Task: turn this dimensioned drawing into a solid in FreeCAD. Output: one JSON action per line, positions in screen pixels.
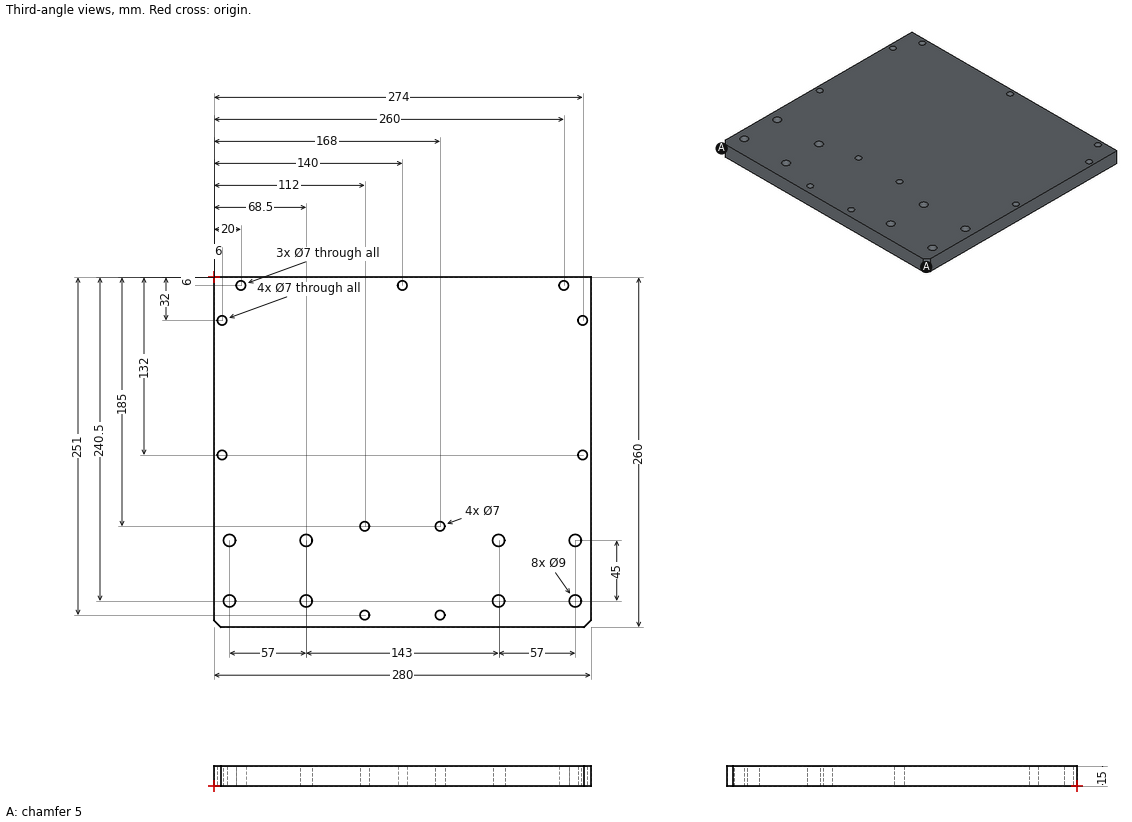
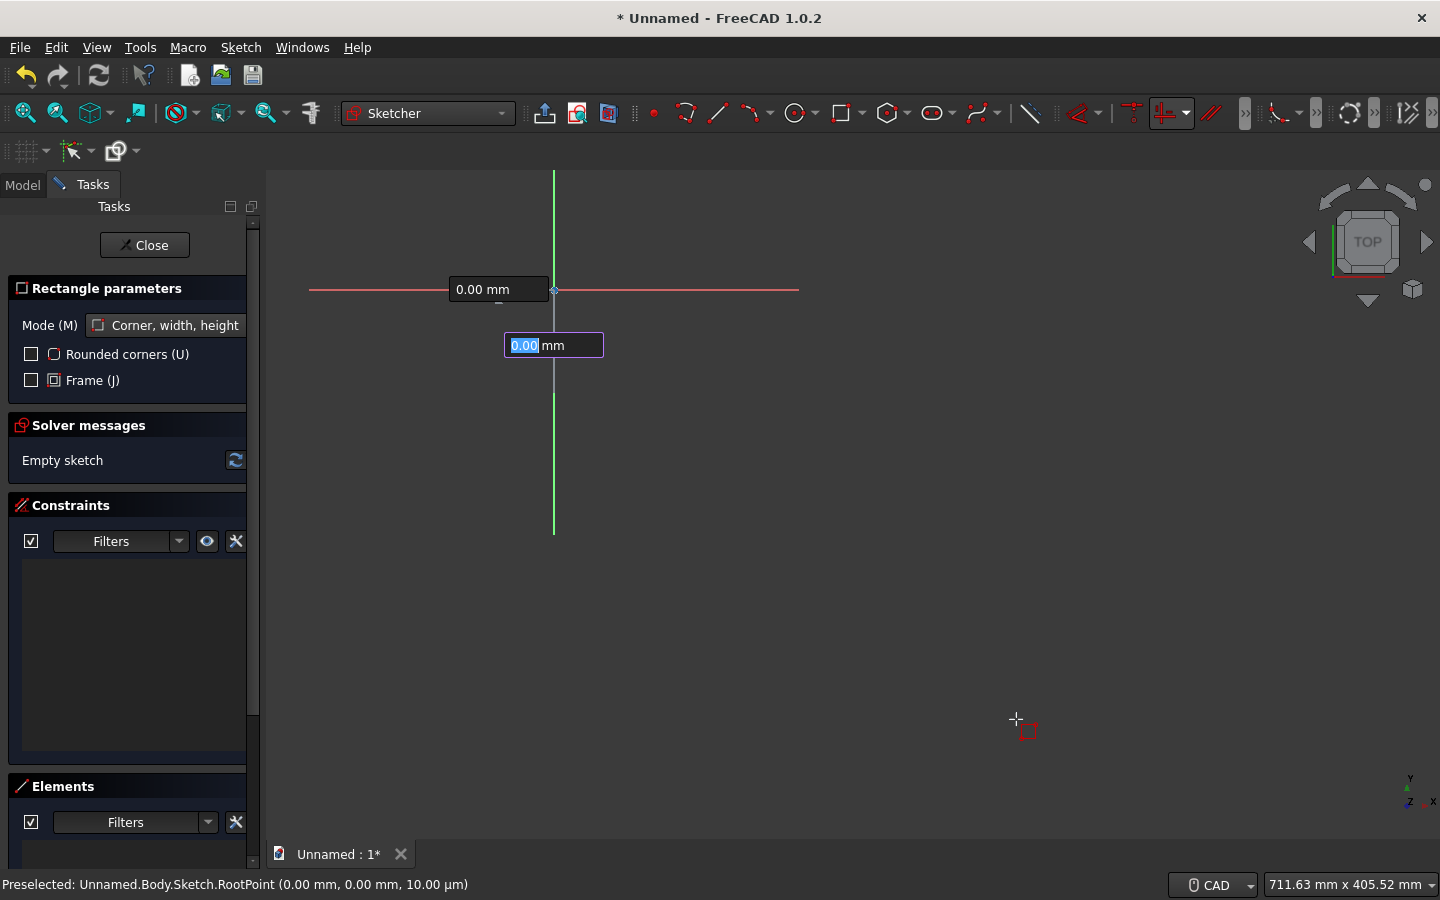
{"action": "type", "text": "280"}
{"action": "key", "text": "Tab"}
{"action": "type", "text": "260"}
{"action": "key", "text": "Return"}
{"action": "key", "text": "Escape"}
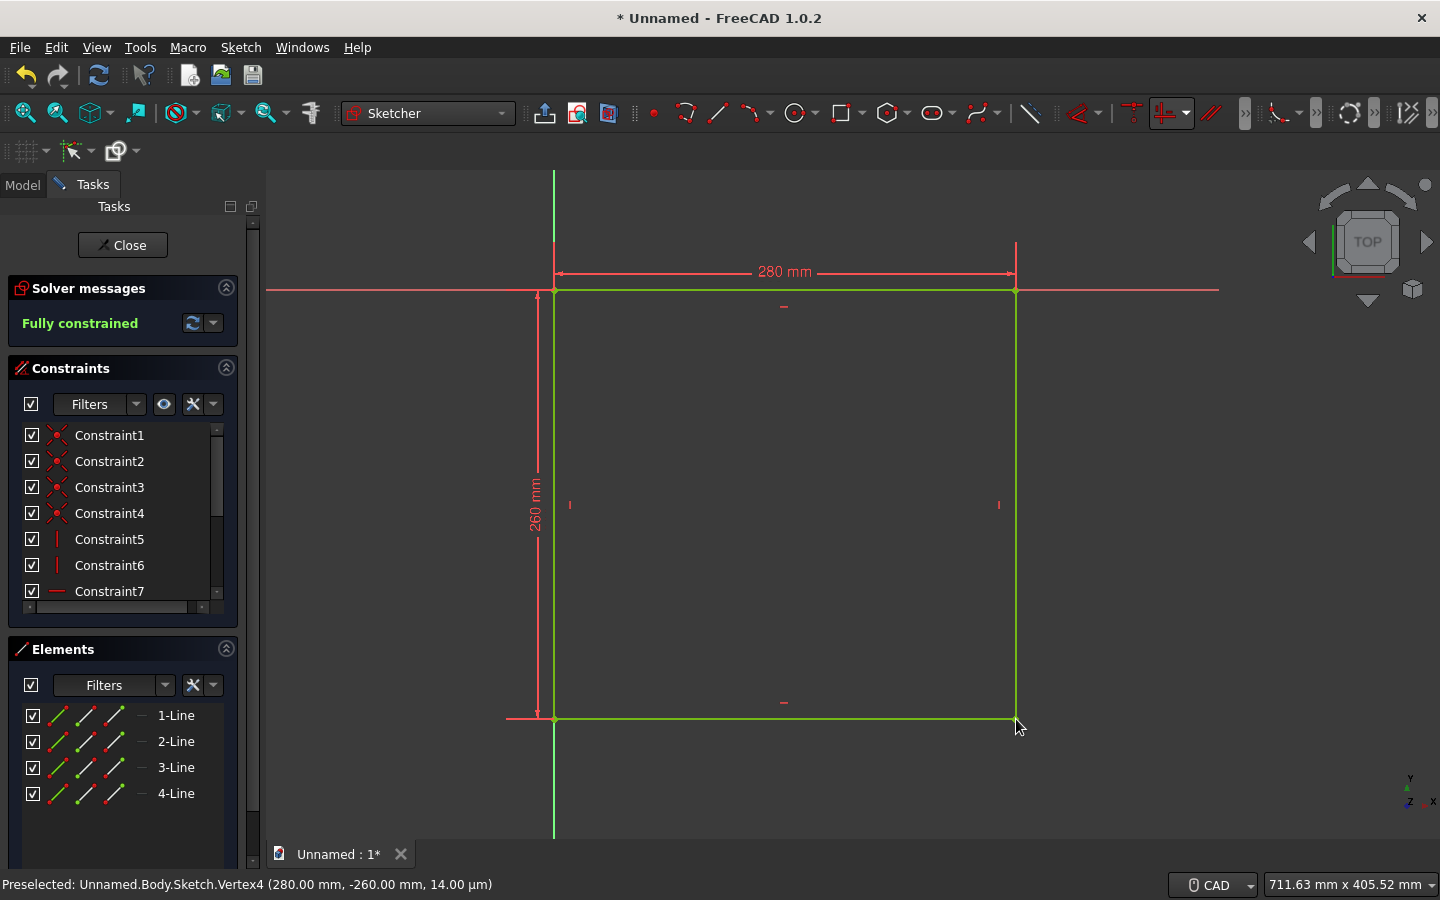
{"action": "left_click", "coordinate": [123, 245]}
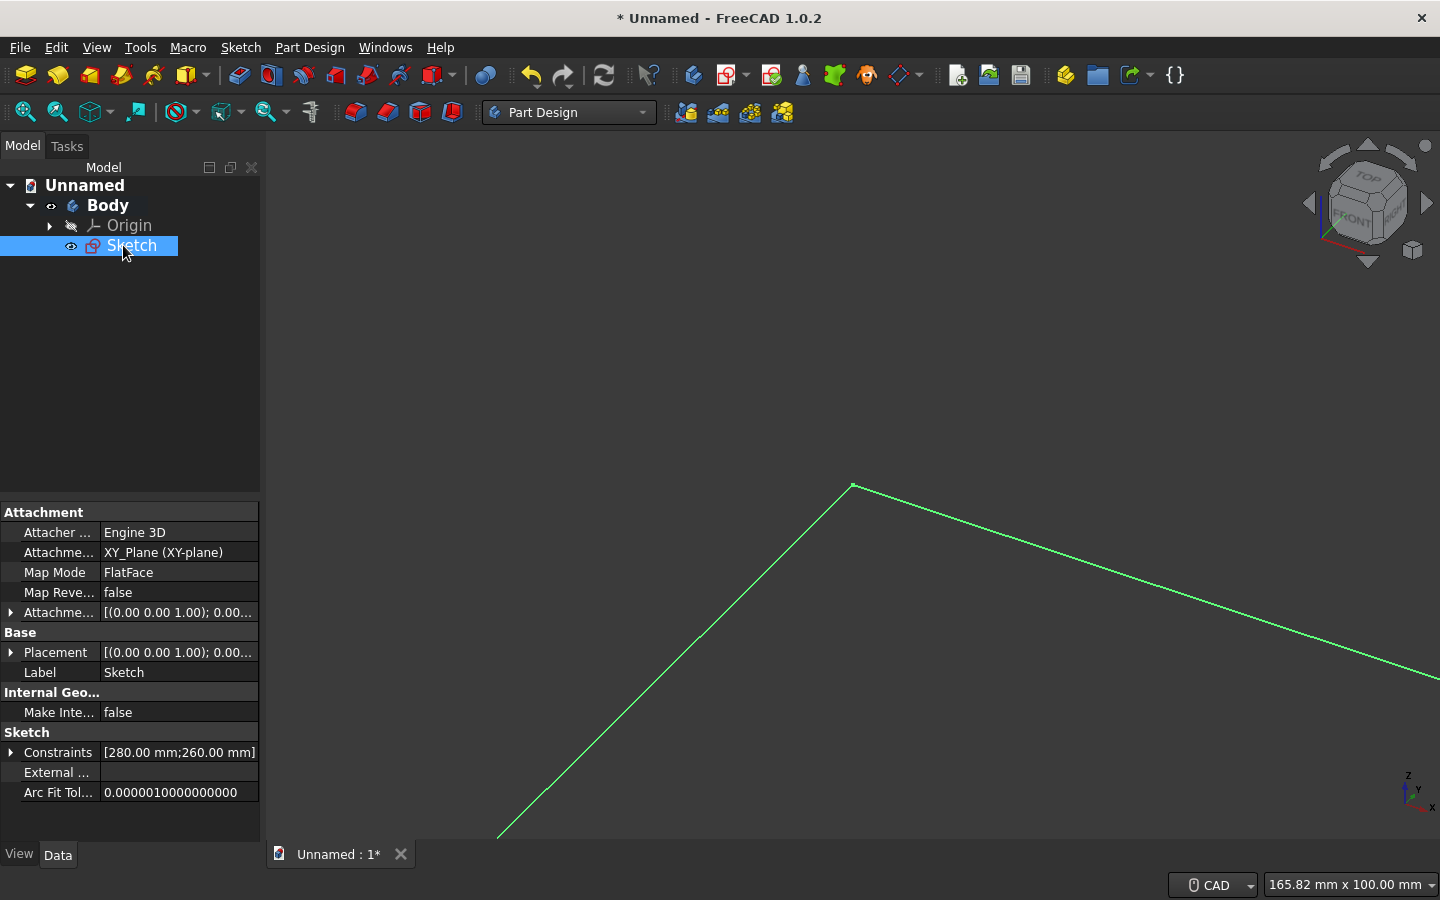
{"action": "left_click", "coordinate": [26, 76]}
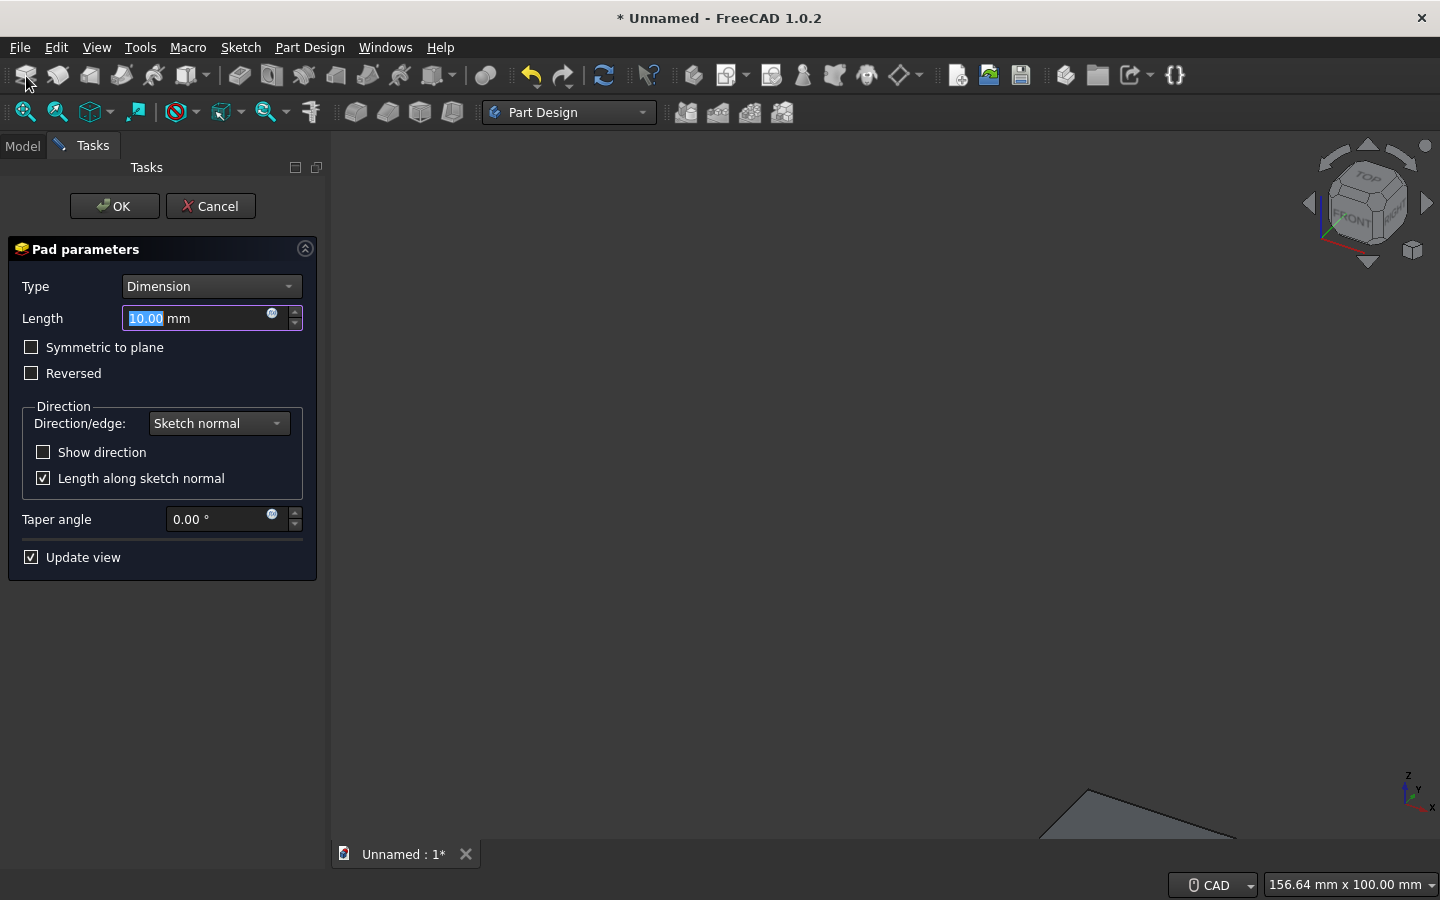
{"action": "type", "text": "15"}
{"action": "key", "text": "Tab"}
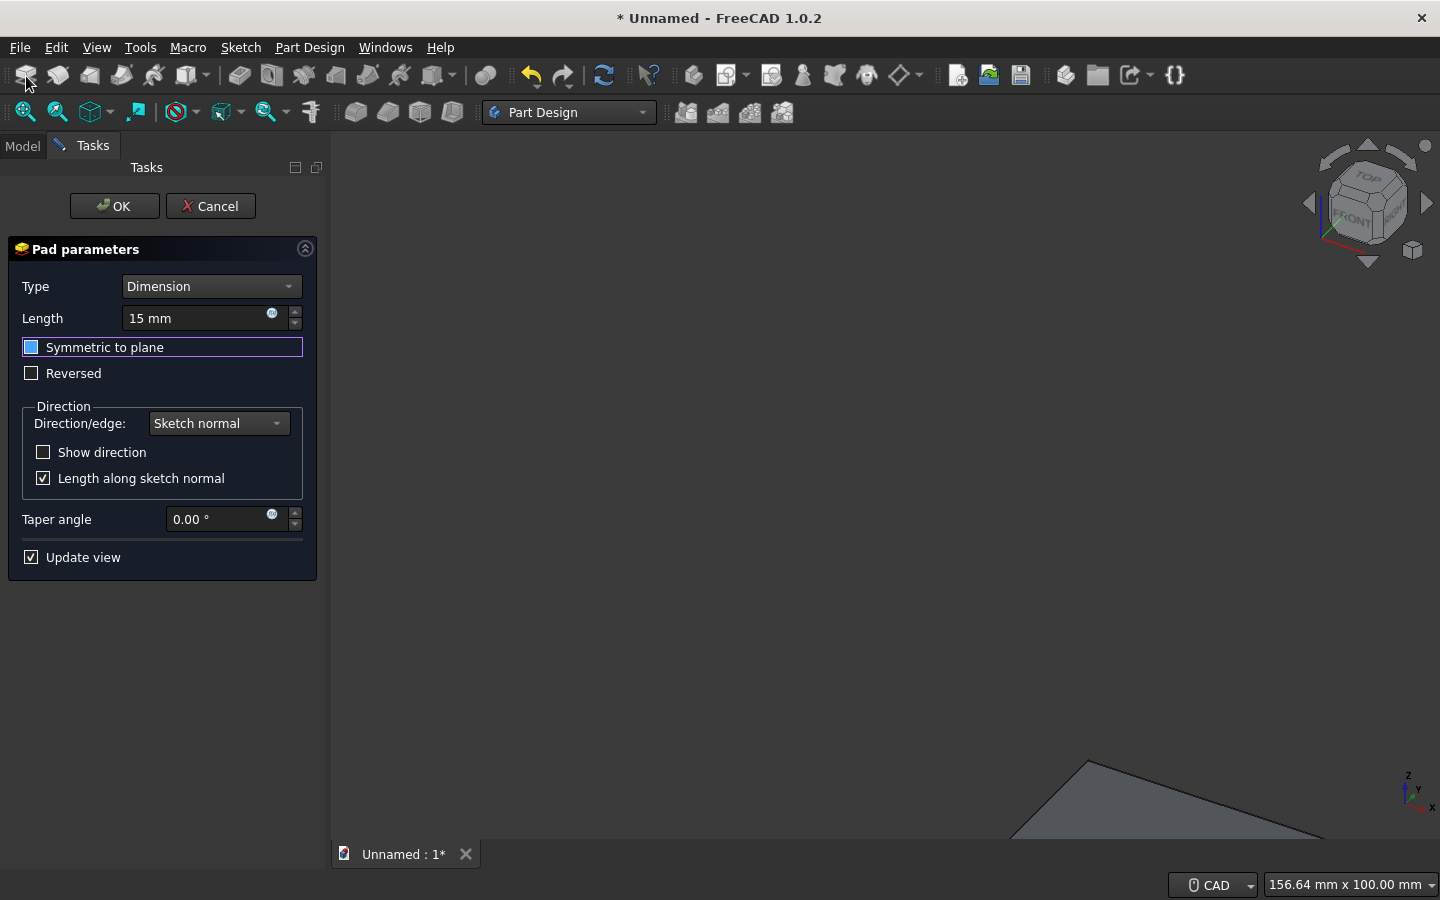
{"action": "left_click", "coordinate": [115, 206]}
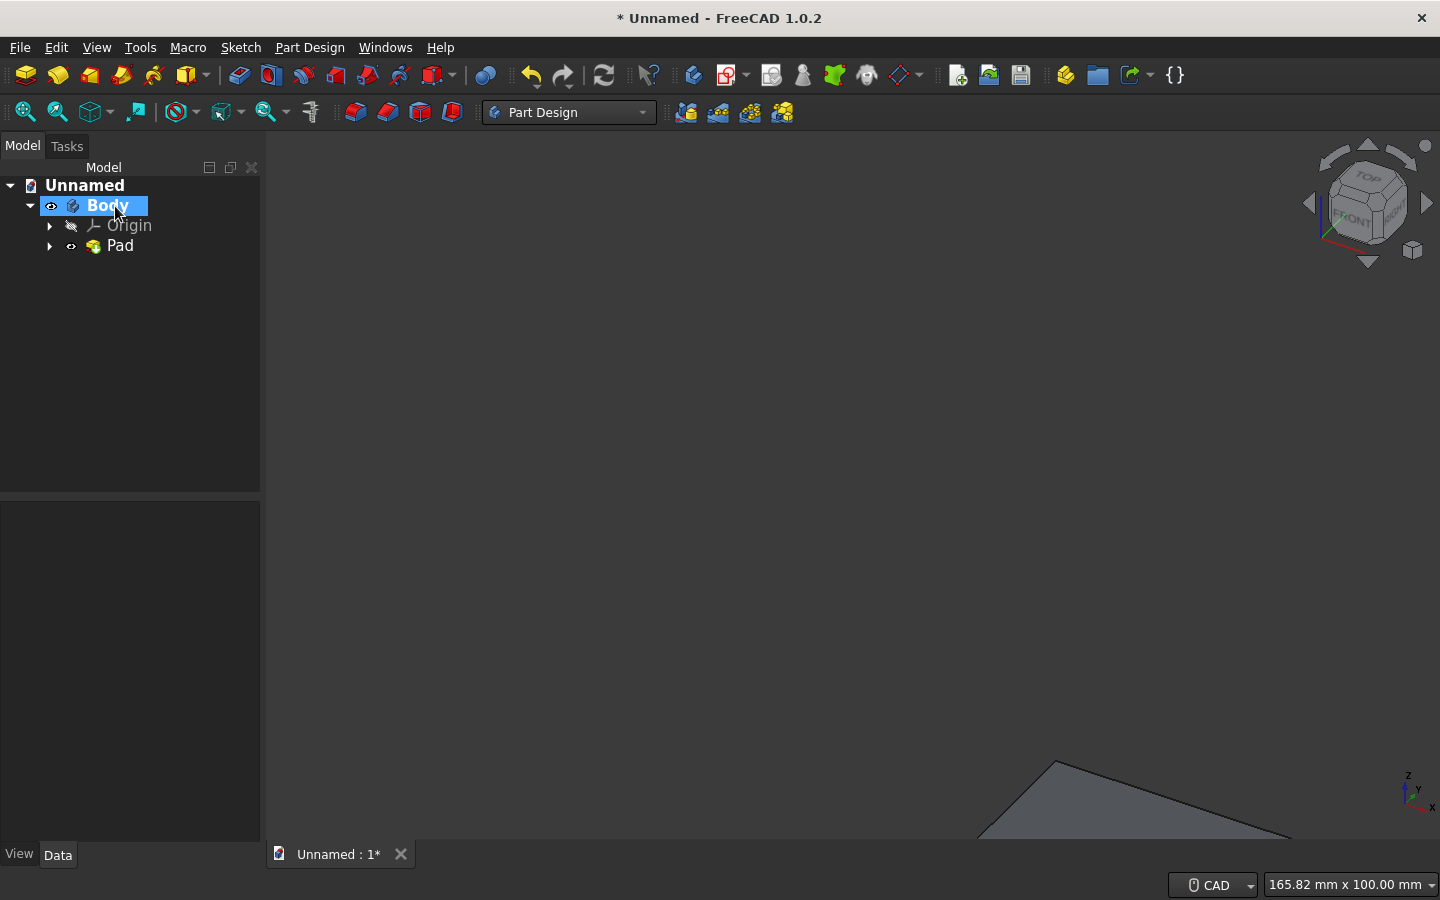
{"action": "left_click", "coordinate": [26, 112]}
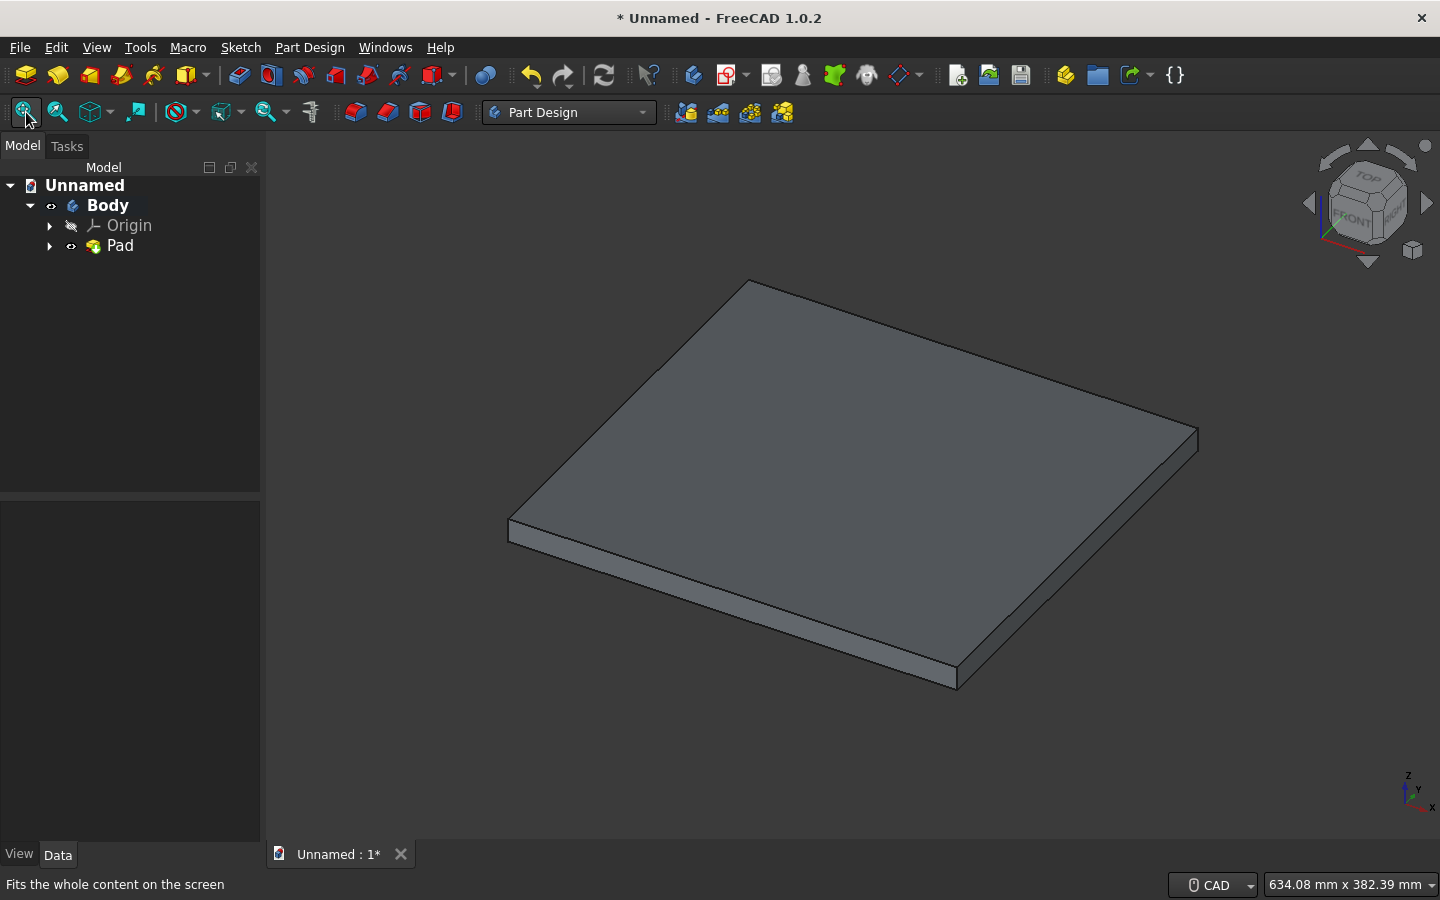
{"action": "left_click", "coordinate": [957, 678]}